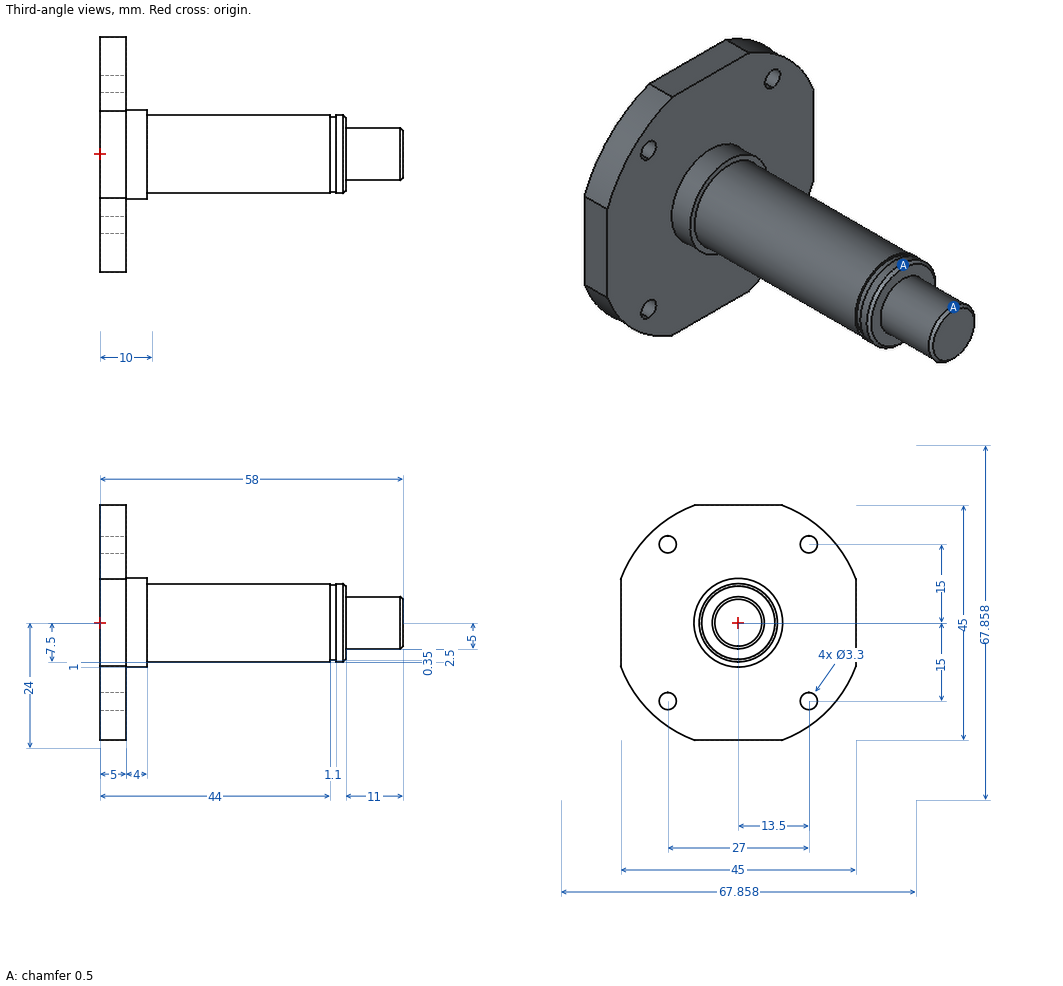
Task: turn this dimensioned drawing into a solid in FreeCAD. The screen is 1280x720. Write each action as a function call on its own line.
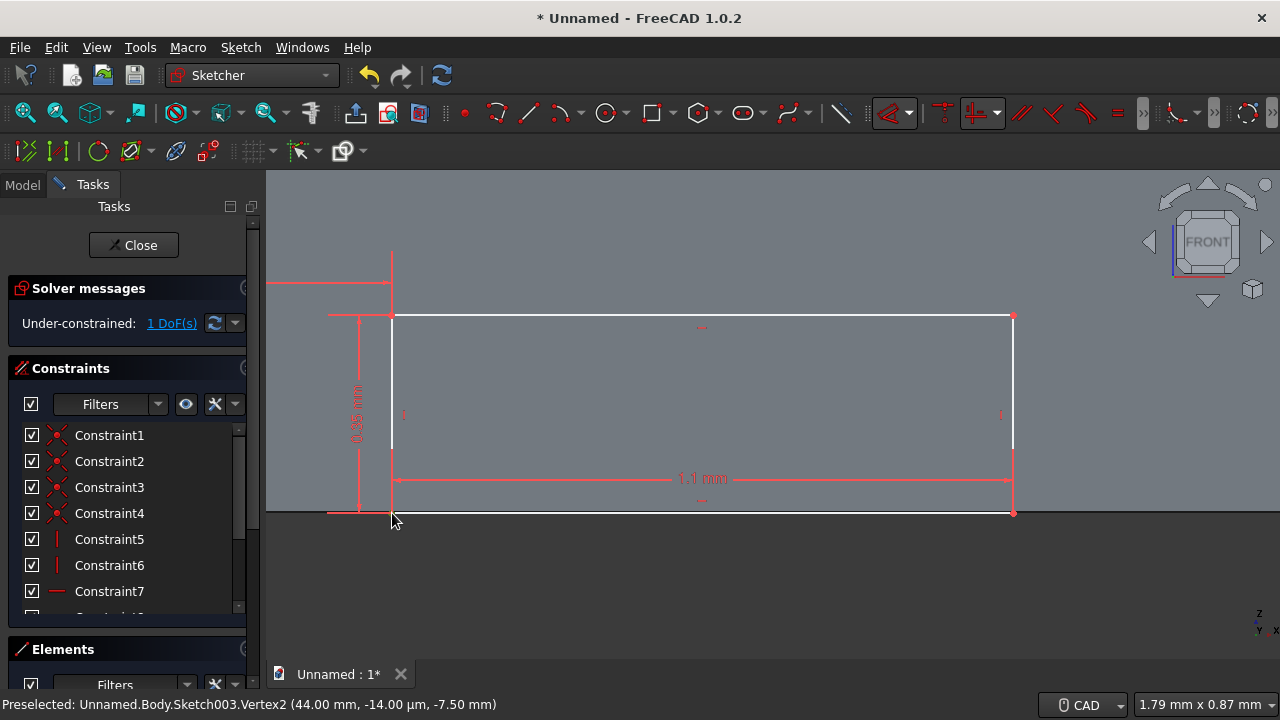
key(i)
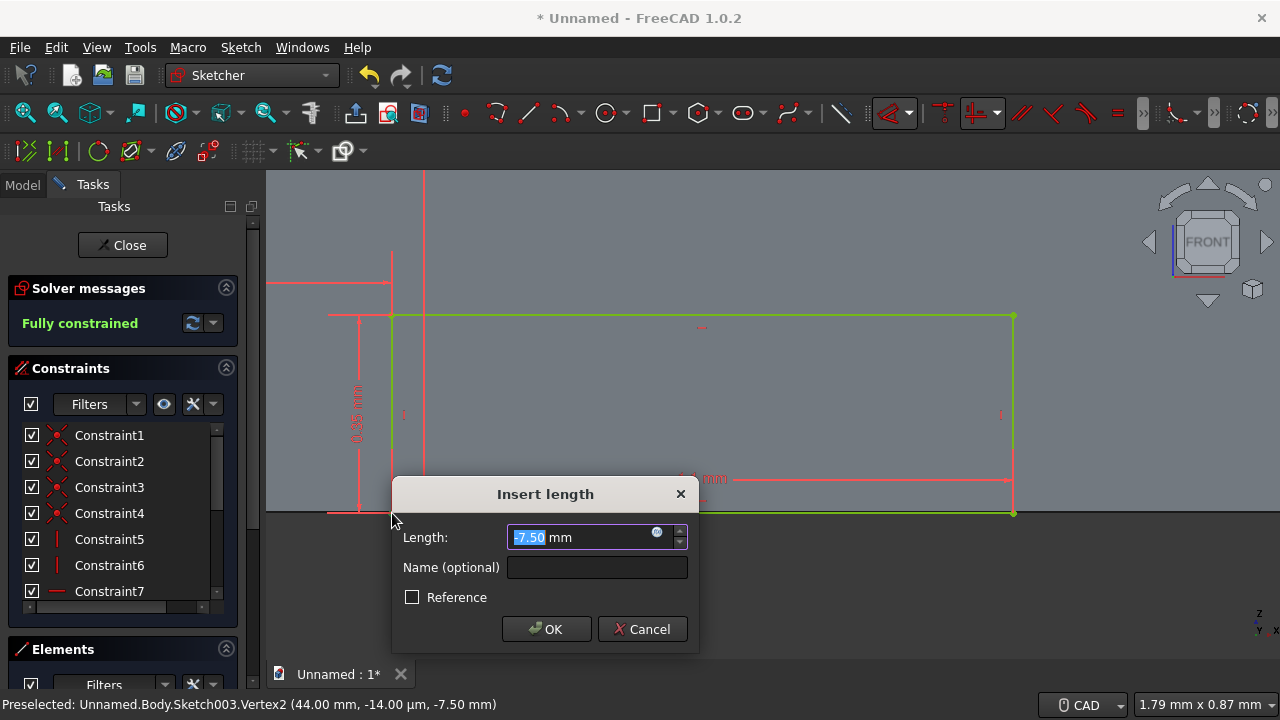
text(-7.5)
key(Return)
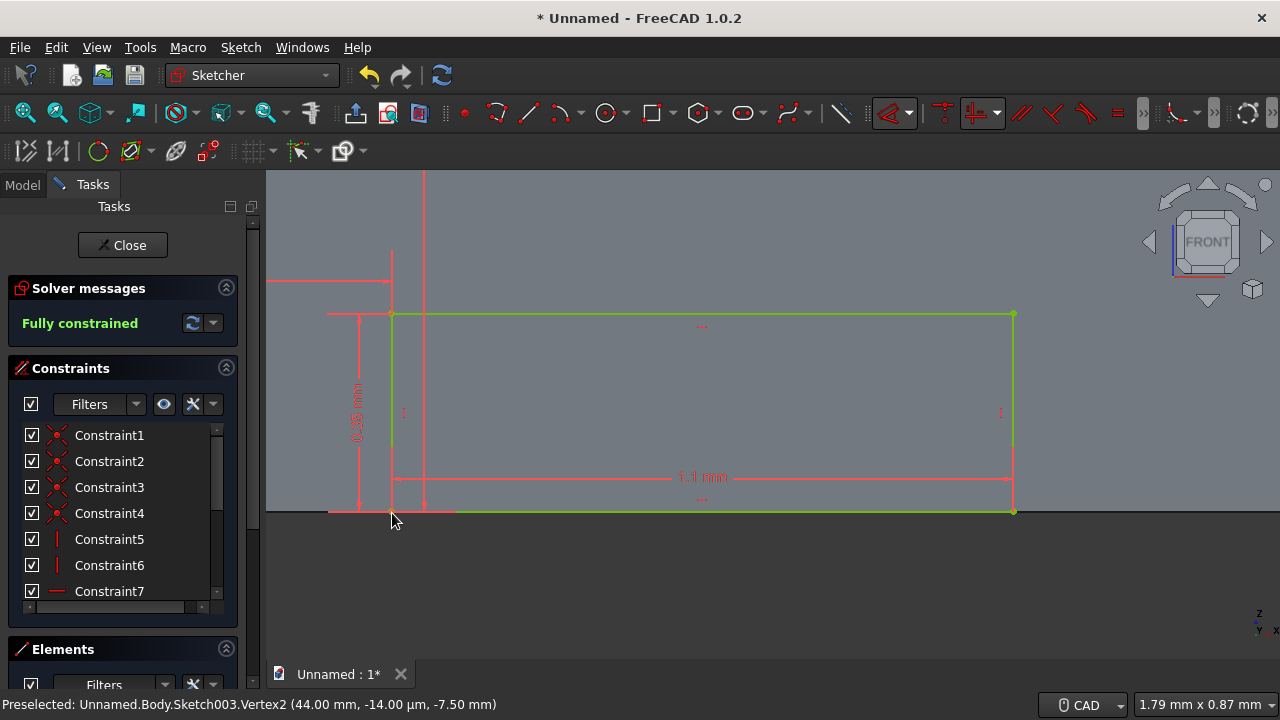
click(123, 245)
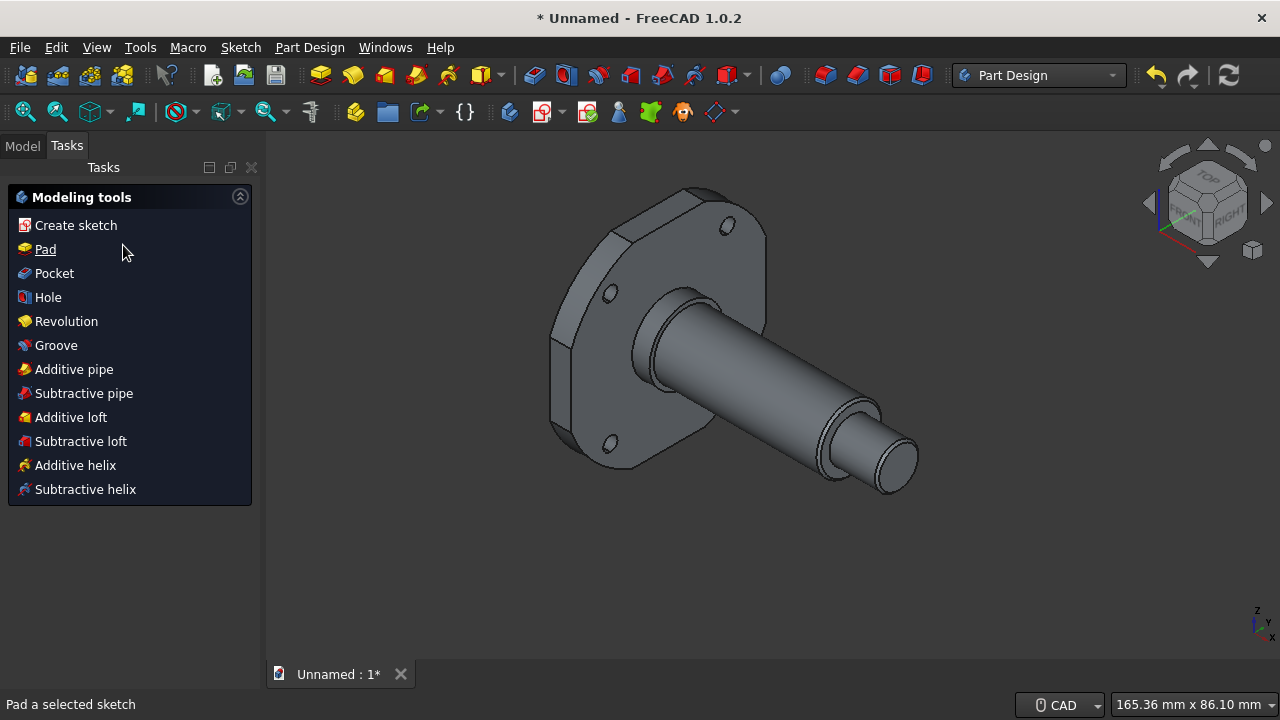
click(600, 76)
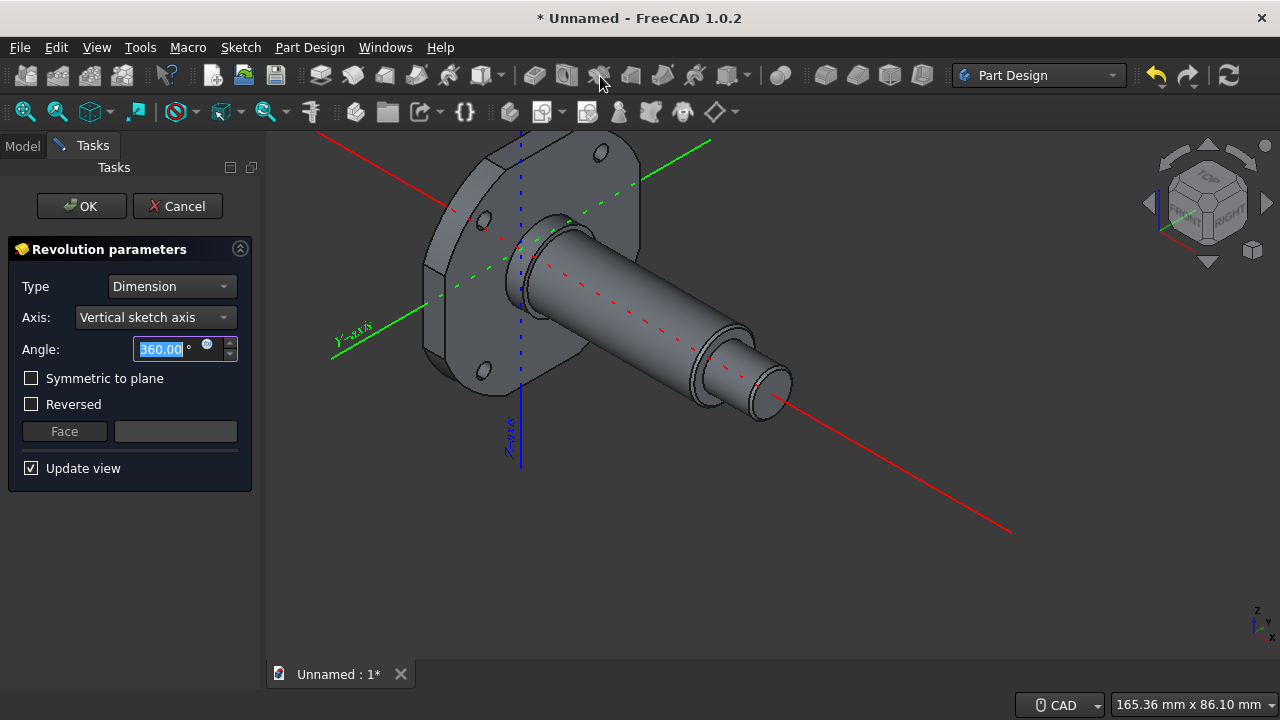
click(156, 318)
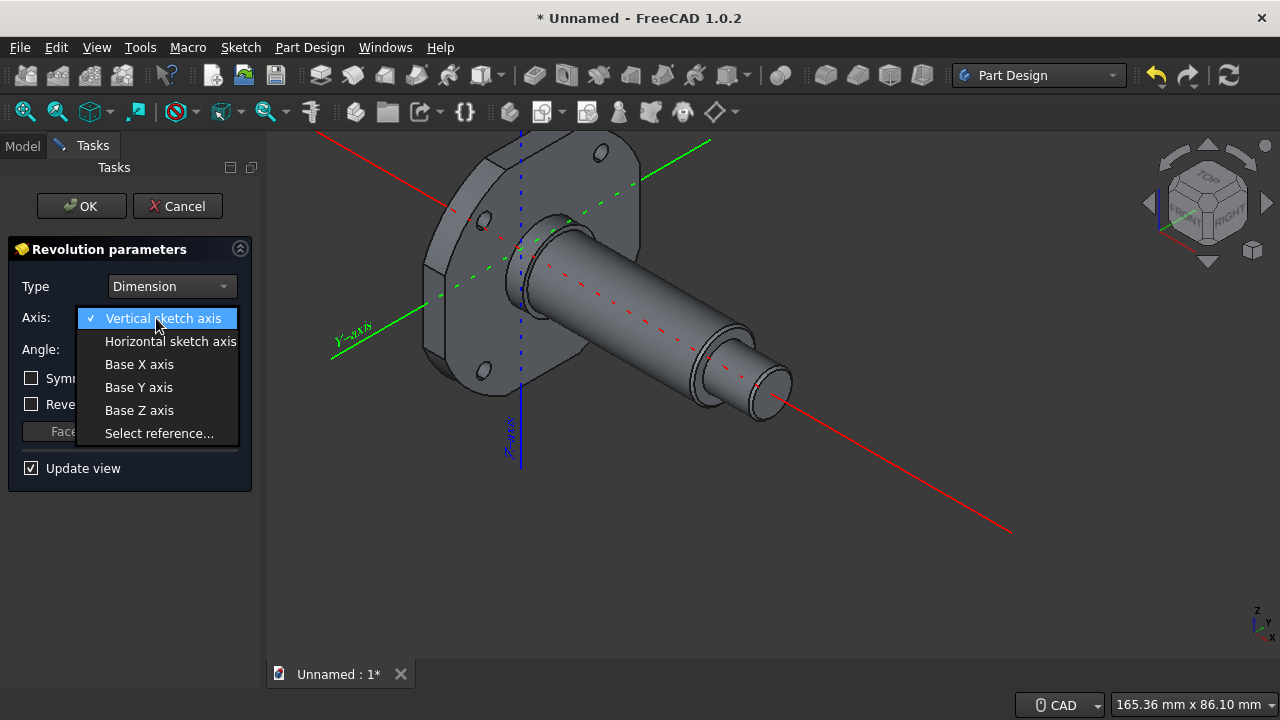
click(156, 342)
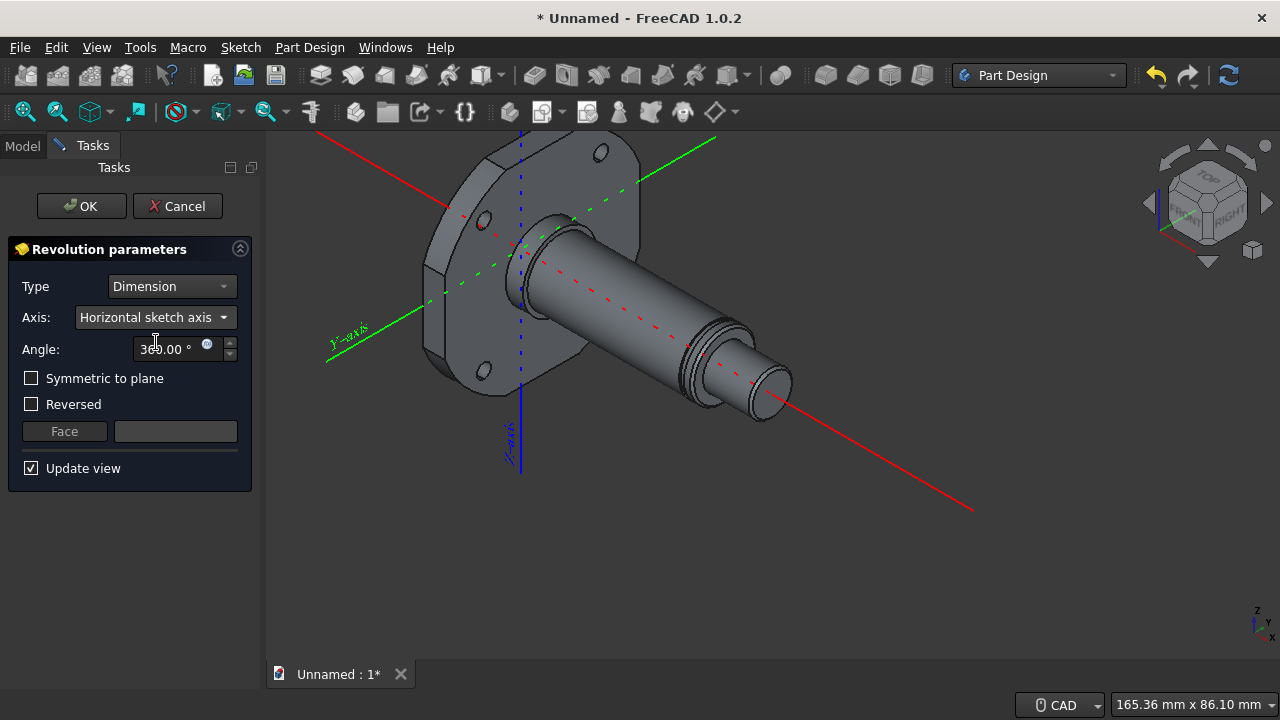
click(82, 206)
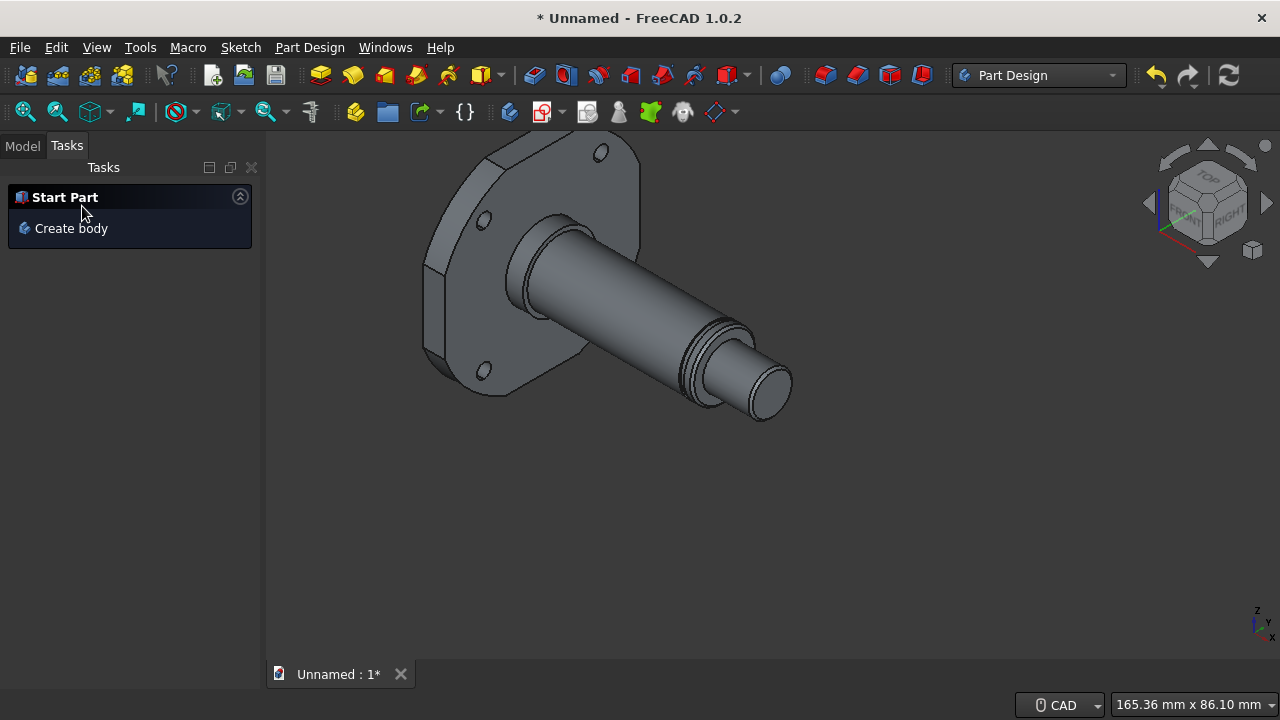
click(26, 112)